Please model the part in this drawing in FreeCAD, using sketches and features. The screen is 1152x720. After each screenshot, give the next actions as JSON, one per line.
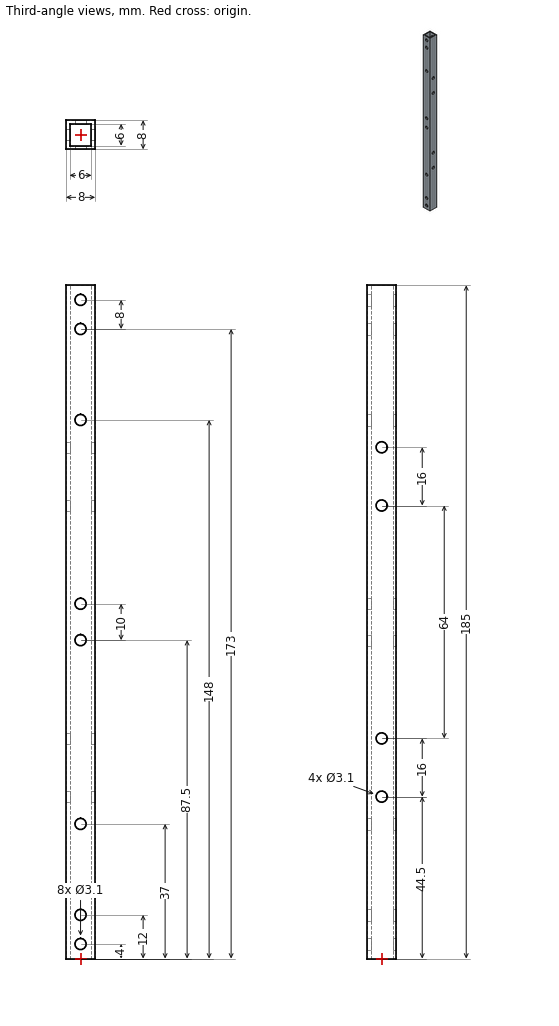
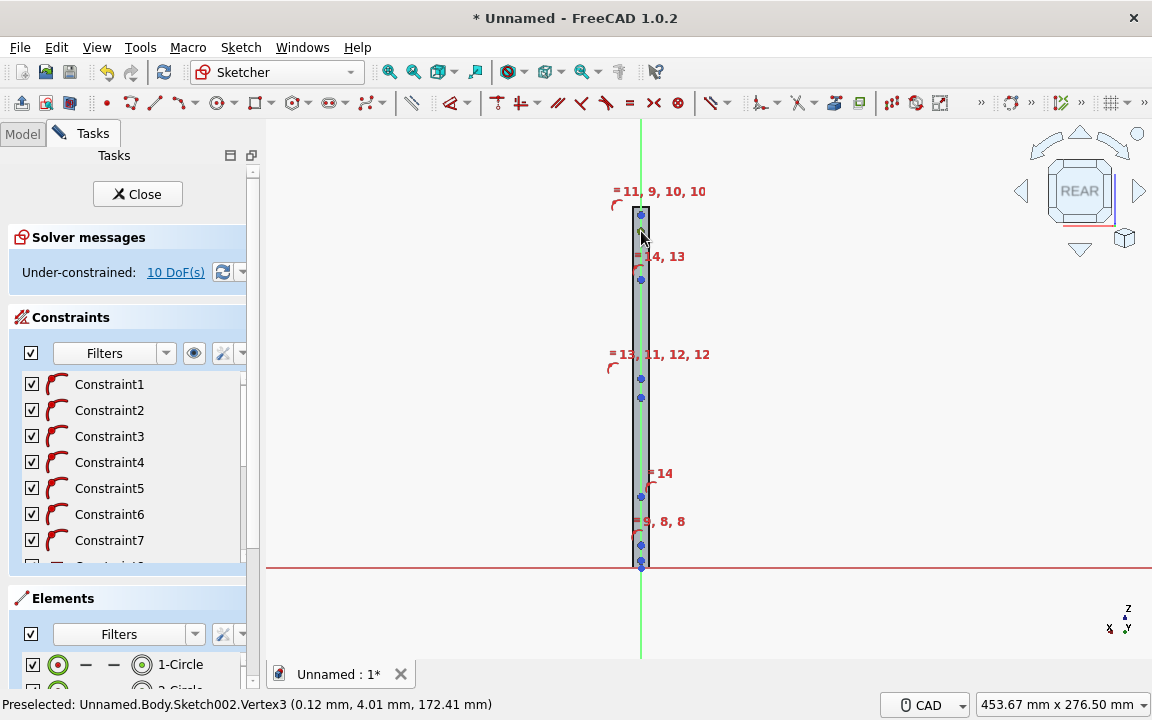
{"action": "left_click", "coordinate": [641, 458]}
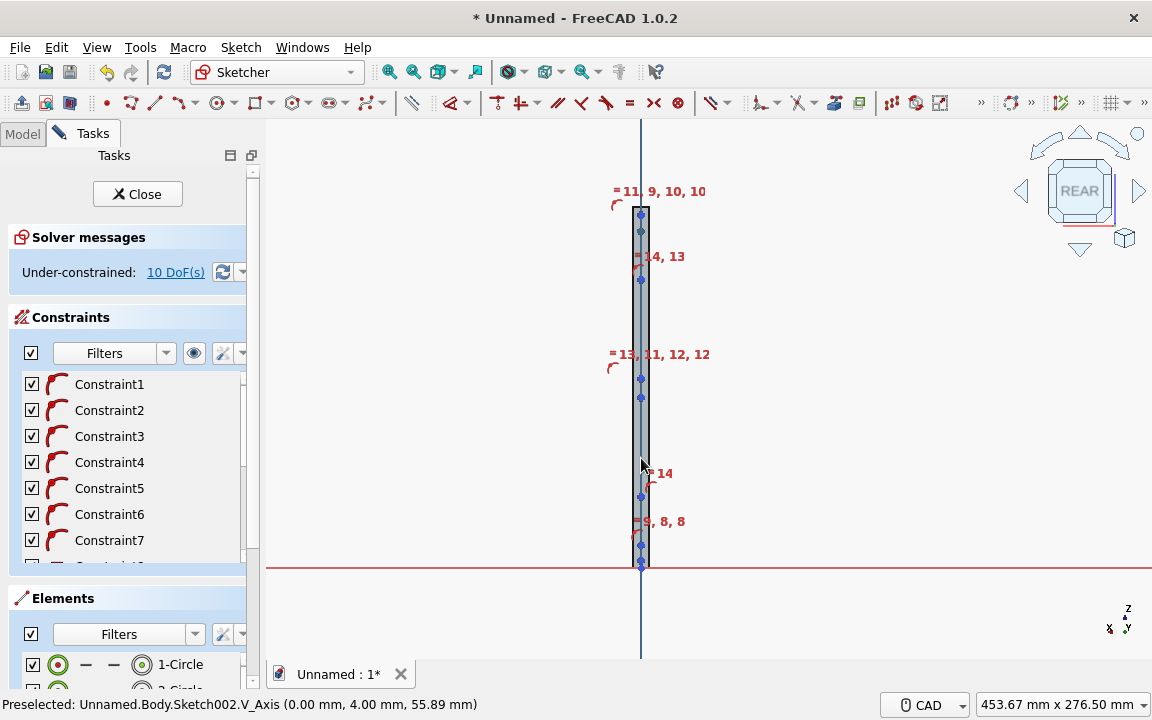
{"action": "left_click", "coordinate": [498, 104]}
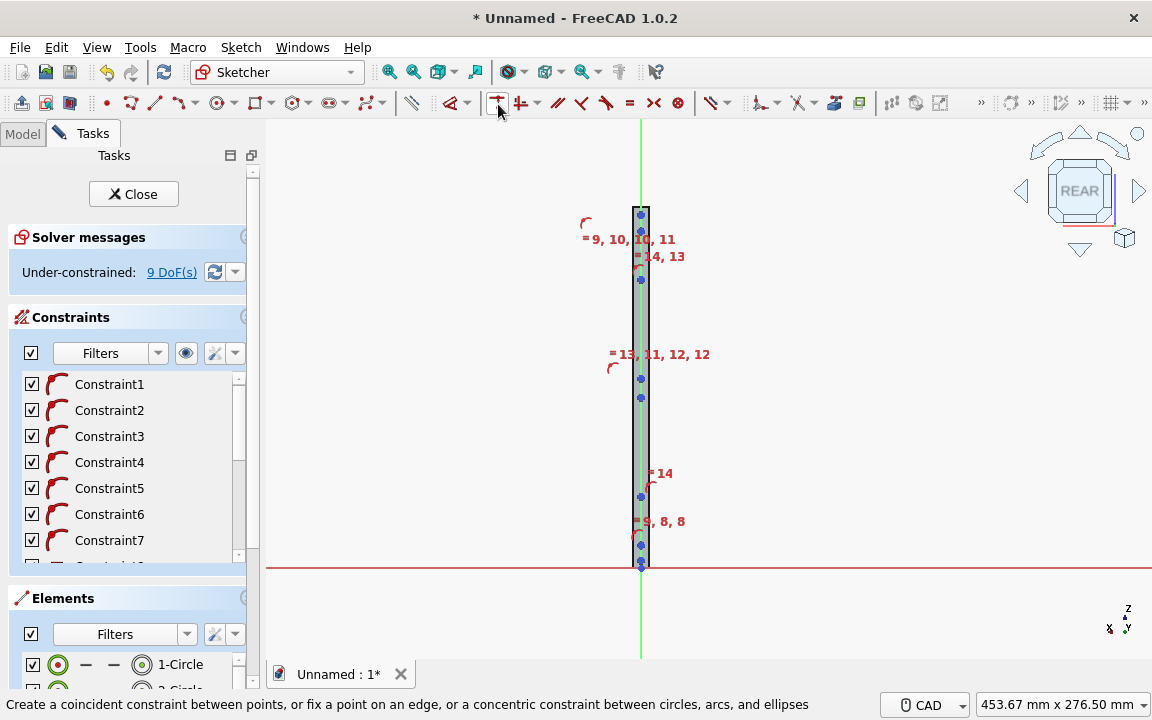
{"action": "left_click", "coordinate": [450, 104]}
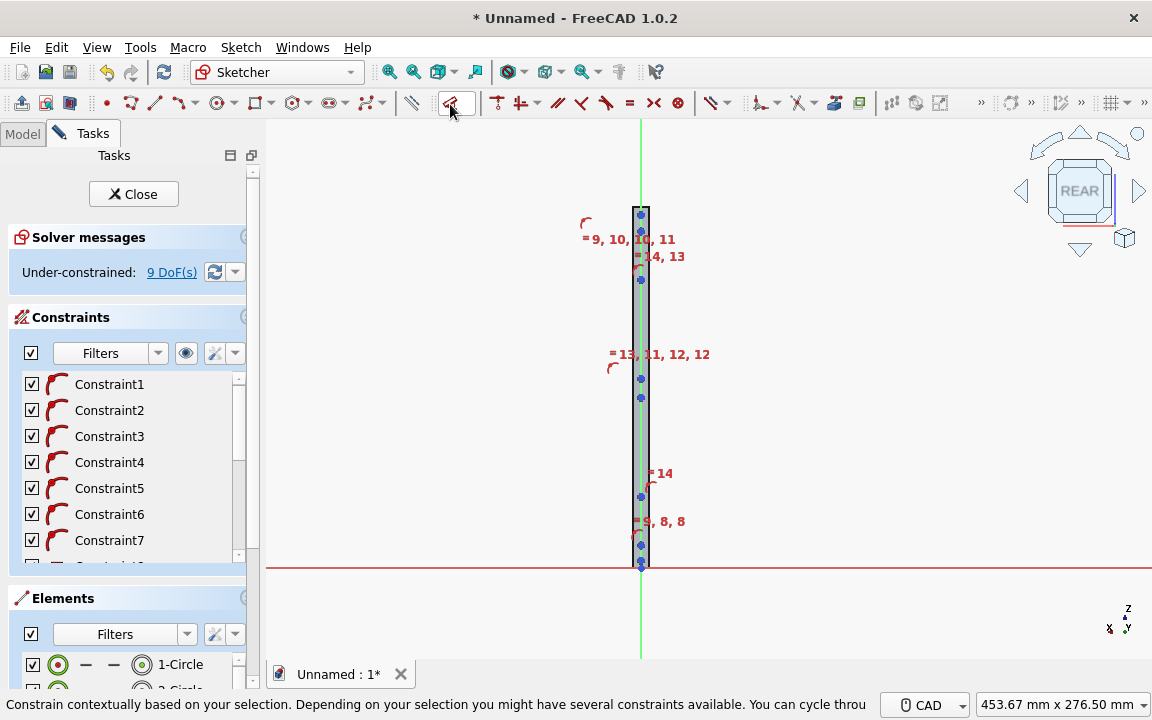
{"action": "scroll", "coordinate": [641, 558], "scroll_direction": "up", "scroll_amount": 10}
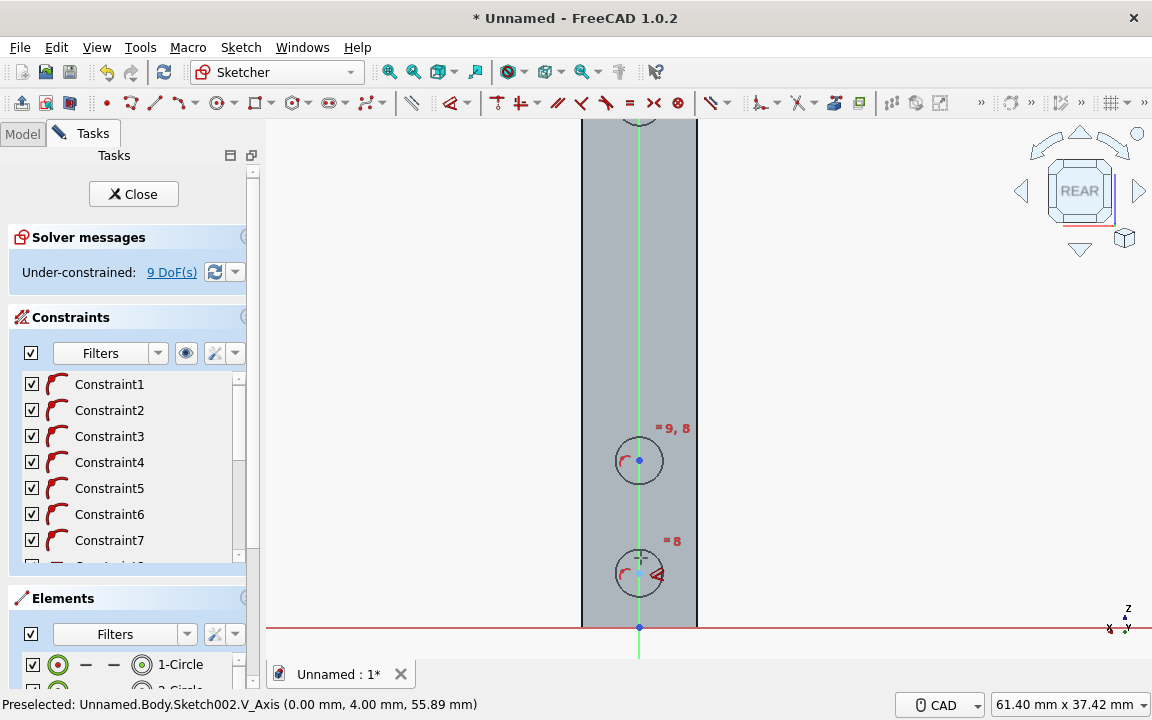
{"action": "left_click", "coordinate": [640, 550]}
{"action": "left_click", "coordinate": [667, 526]}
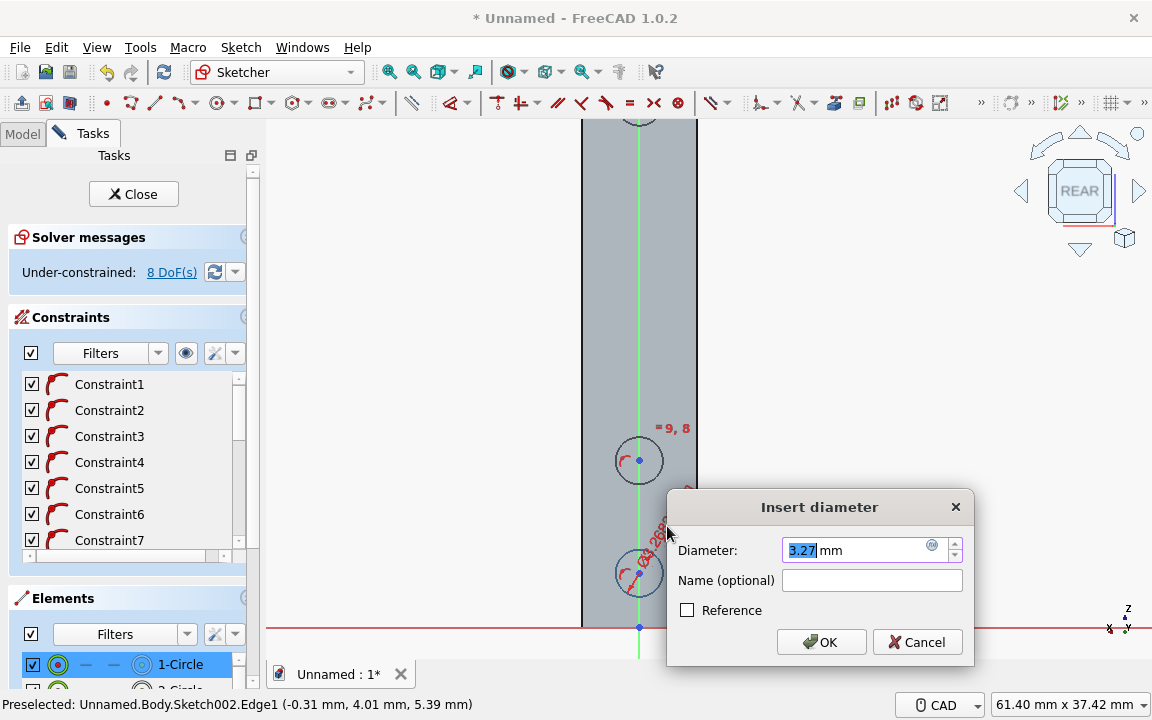
{"action": "type", "text": "3.1"}
{"action": "key", "text": "Return"}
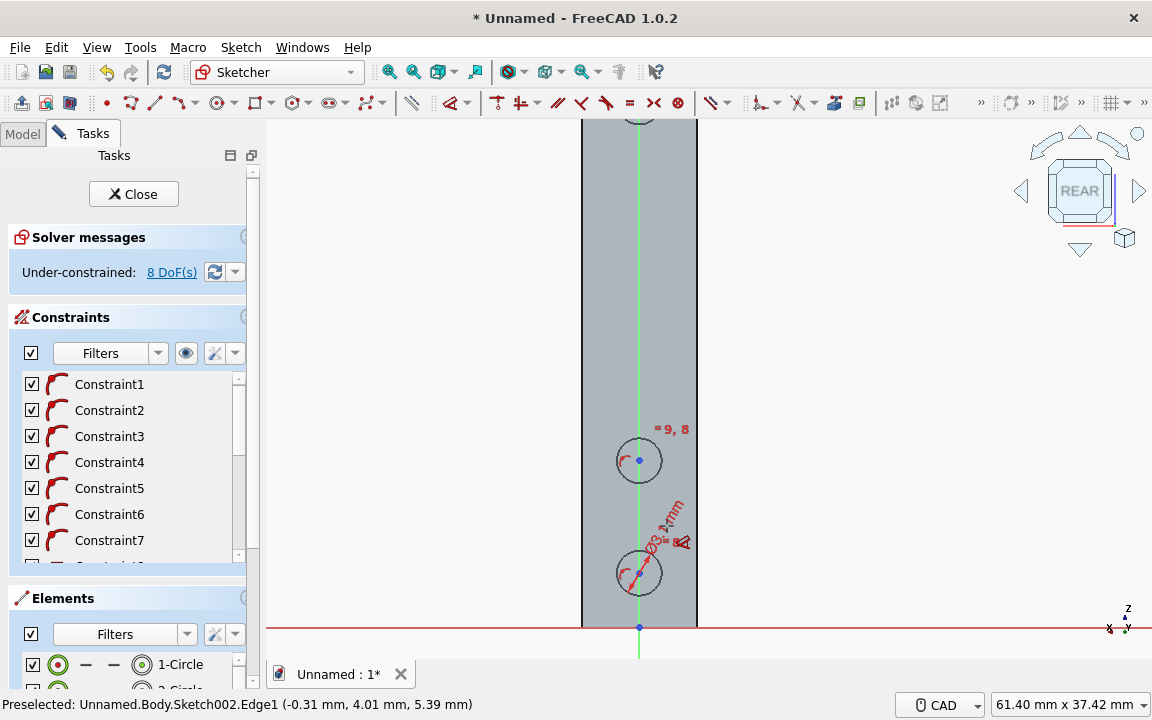
{"action": "left_click", "coordinate": [639, 573]}
{"action": "left_click", "coordinate": [673, 600]}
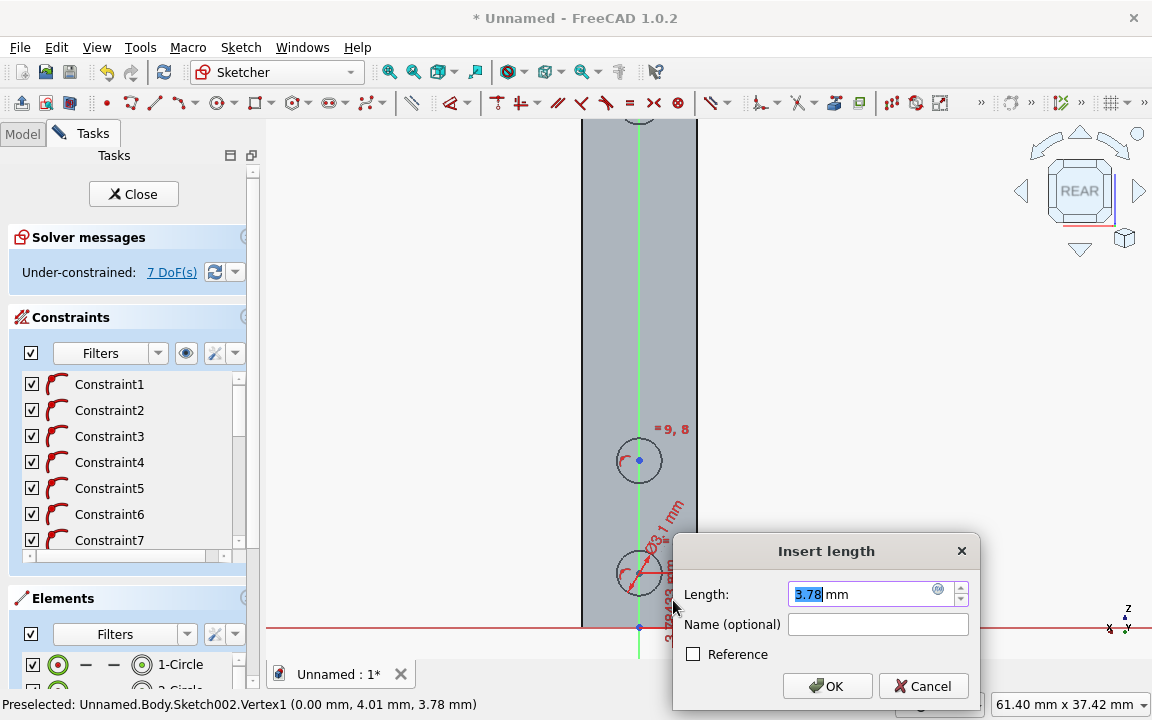
{"action": "type", "text": "4"}
{"action": "key", "text": "Return"}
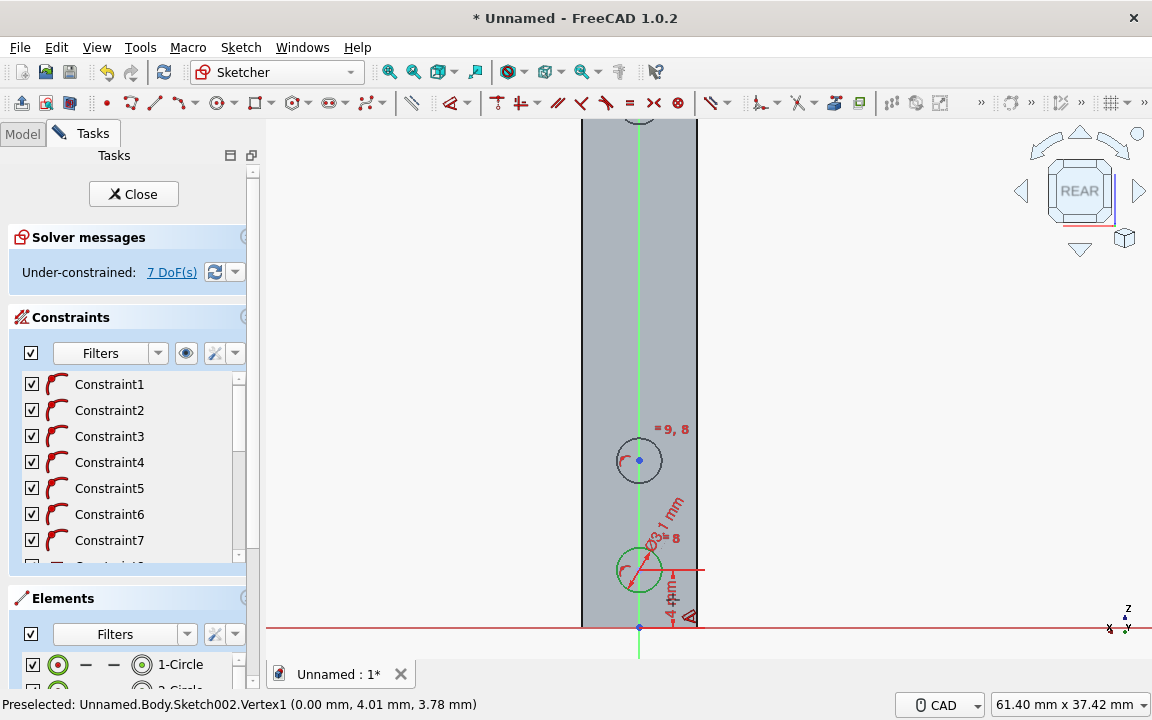
{"action": "scroll", "coordinate": [641, 558], "scroll_direction": "down", "scroll_amount": 10}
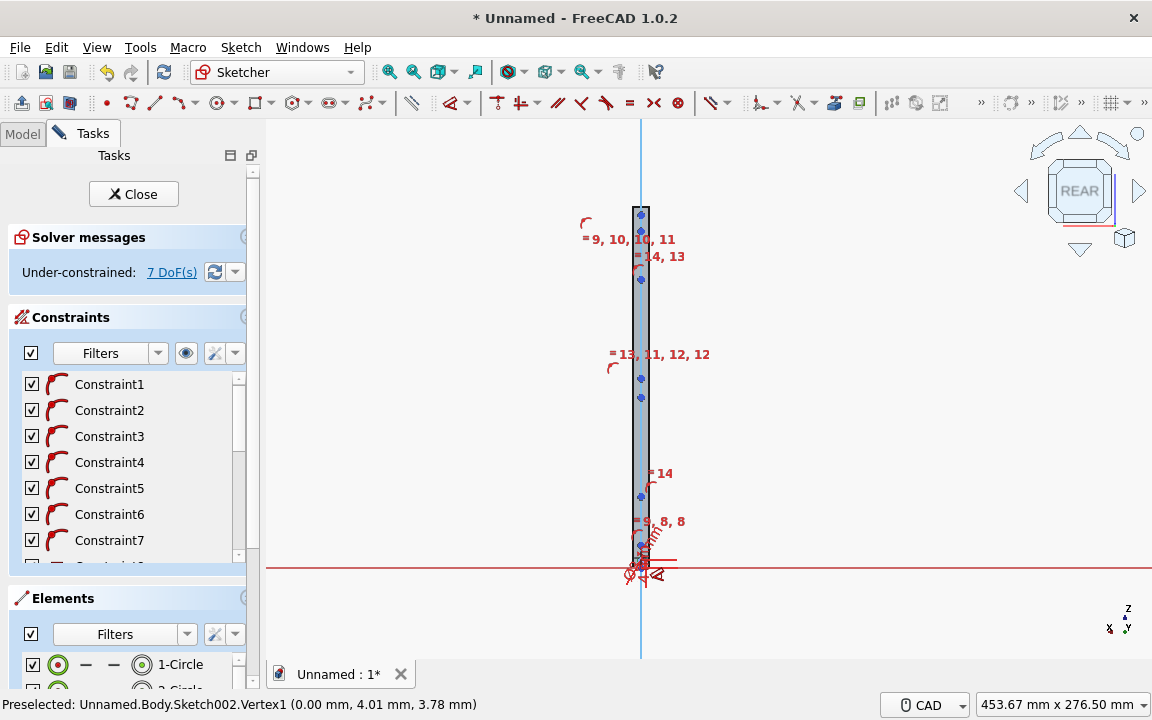
{"action": "scroll", "coordinate": [641, 546], "scroll_direction": "up", "scroll_amount": 3}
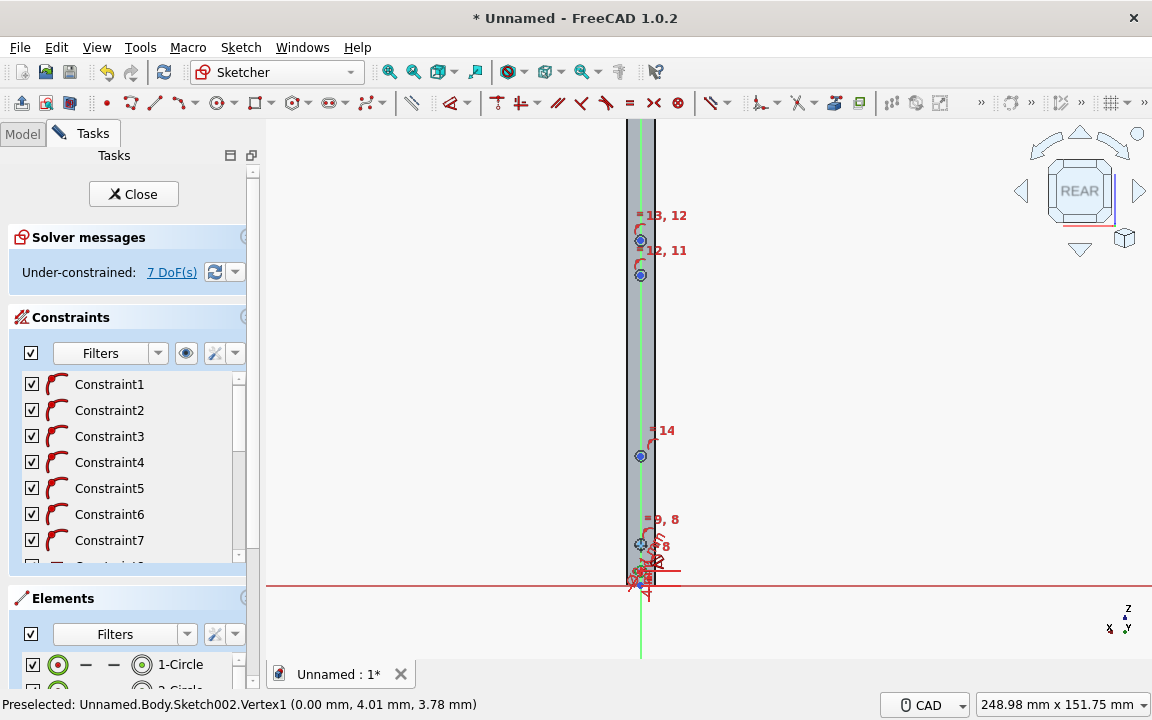
{"action": "left_click", "coordinate": [641, 545]}
{"action": "left_click", "coordinate": [723, 565]}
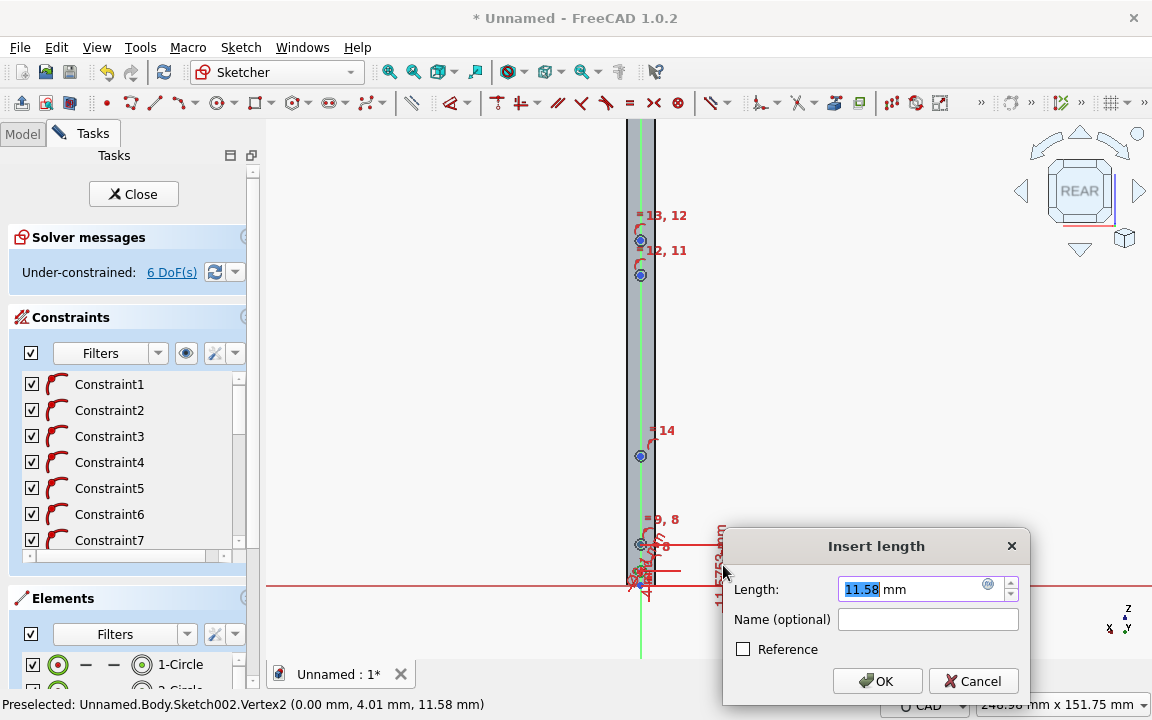
{"action": "type", "text": "12"}
{"action": "key", "text": "Return"}